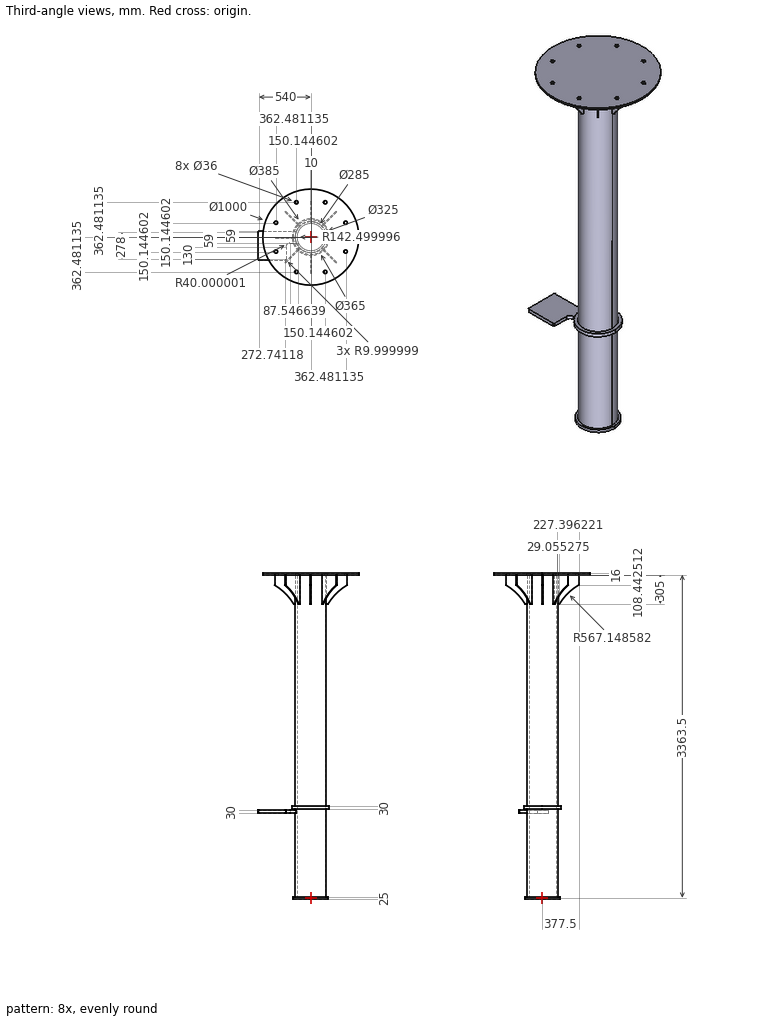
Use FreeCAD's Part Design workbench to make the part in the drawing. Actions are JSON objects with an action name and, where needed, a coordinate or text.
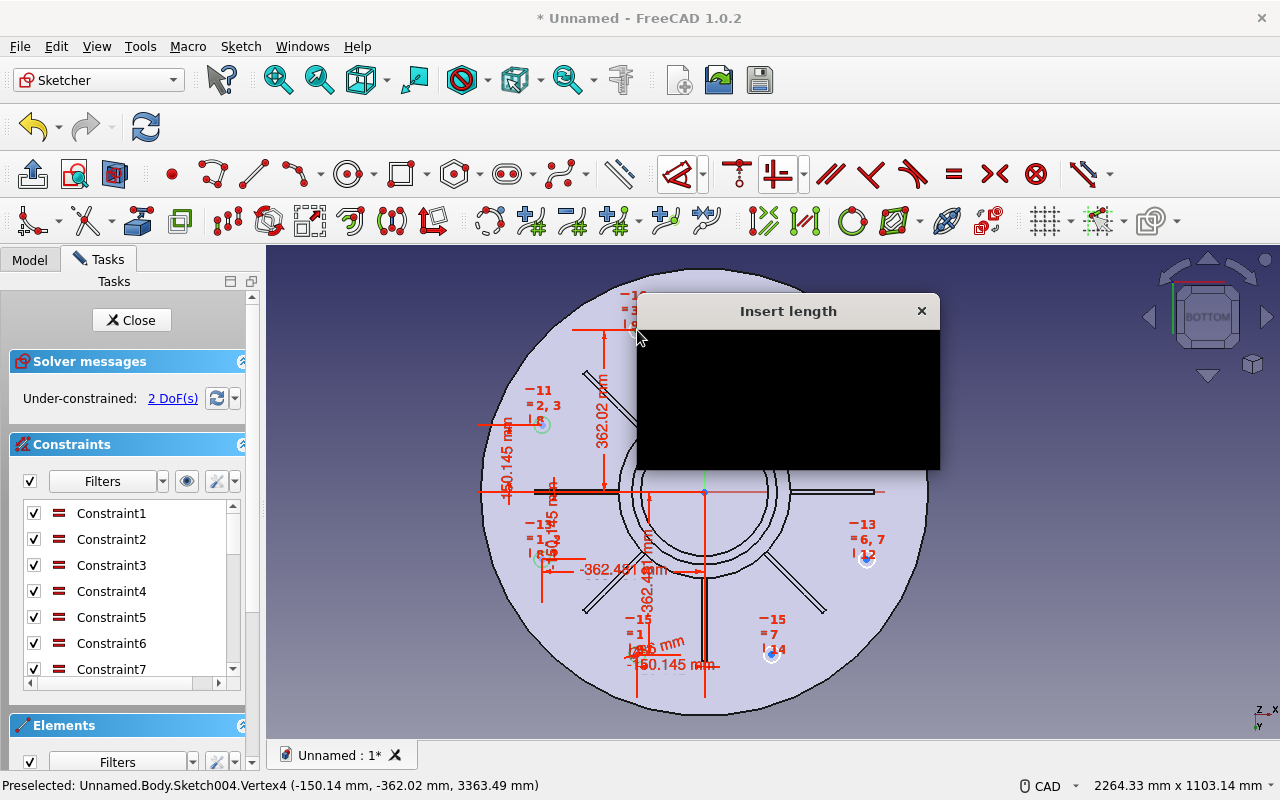
{"action": "type", "text": "362.481135"}
{"action": "key", "text": "Return"}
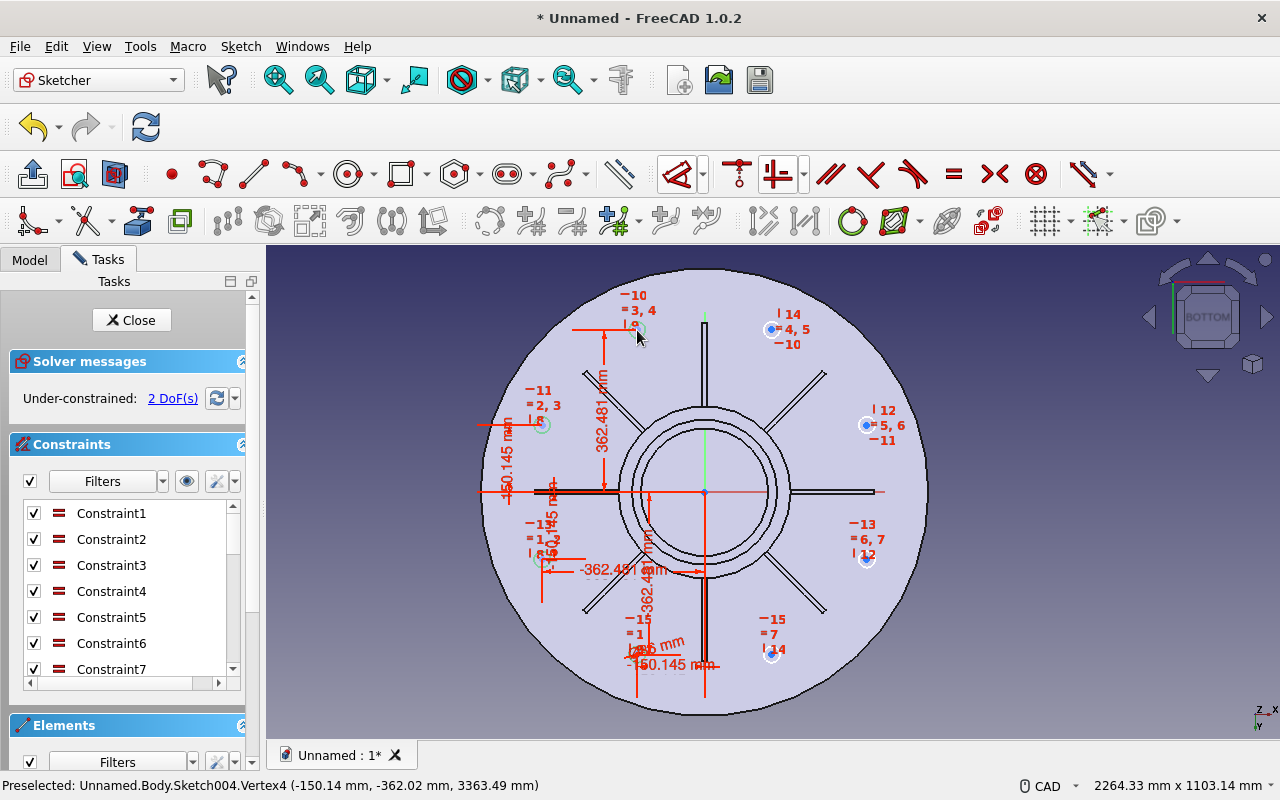
{"action": "left_click", "coordinate": [772, 330]}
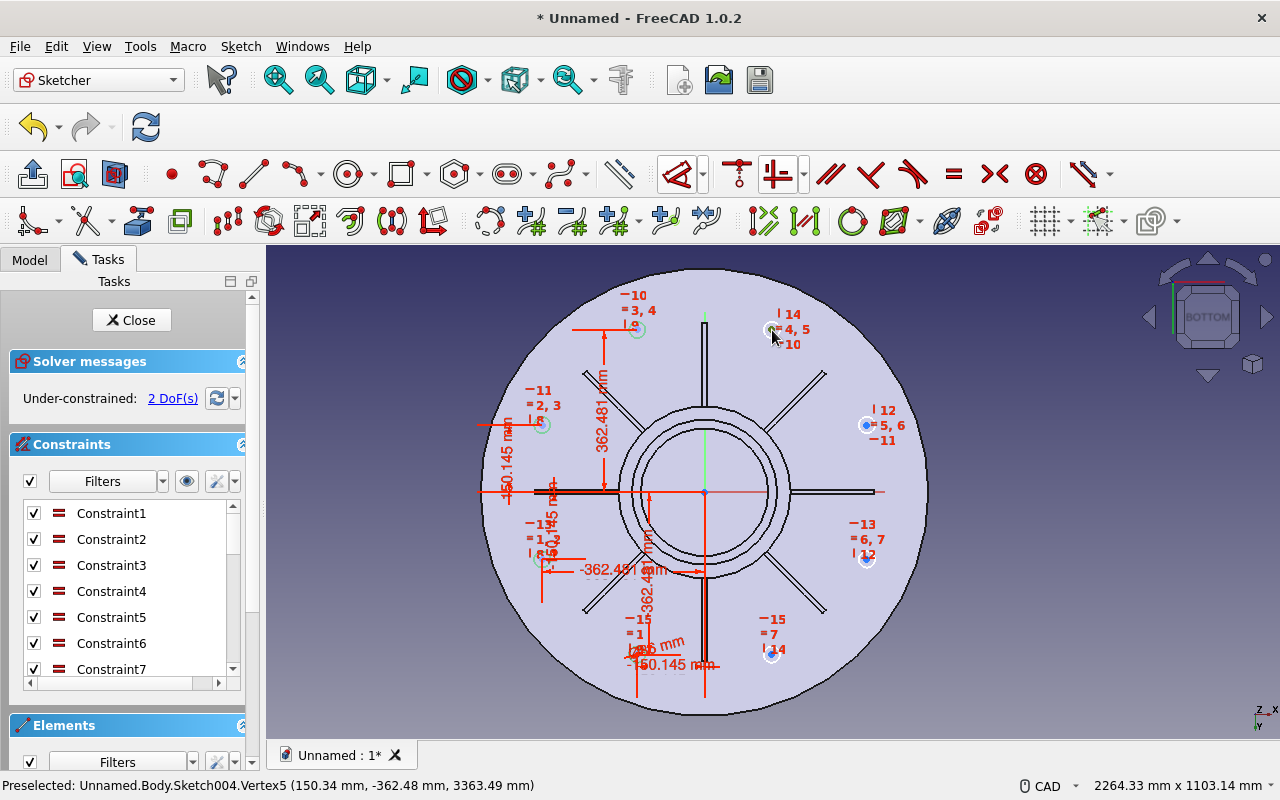
{"action": "left_click", "coordinate": [702, 174]}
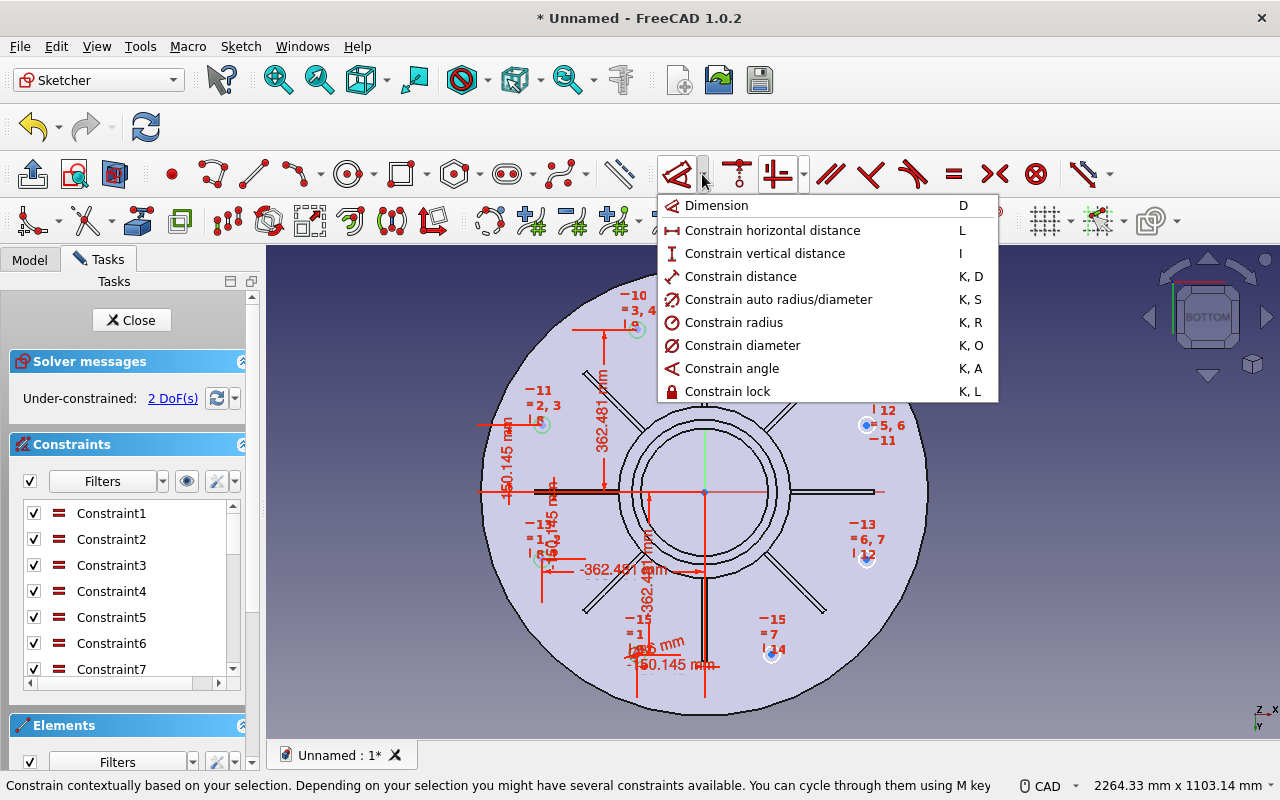
{"action": "left_click", "coordinate": [828, 230]}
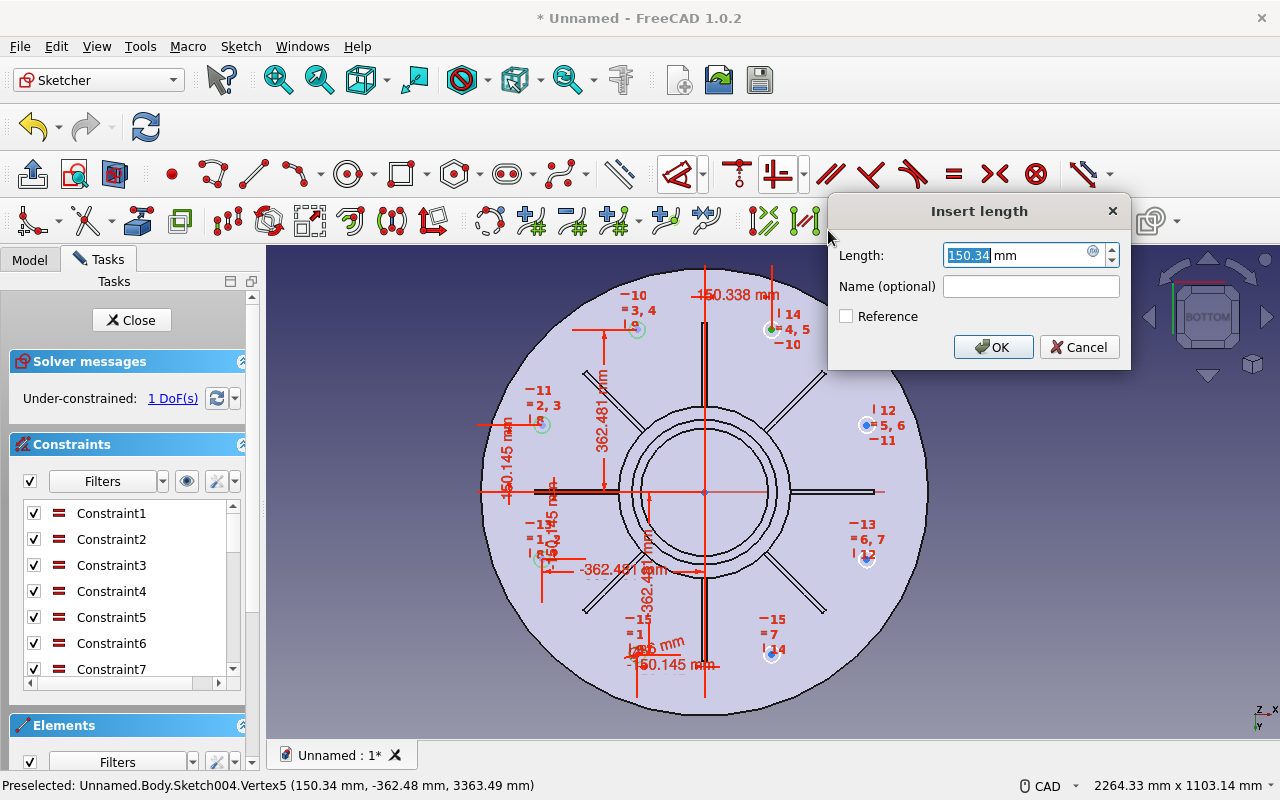
{"action": "type", "text": "150.144602"}
{"action": "key", "text": "Return"}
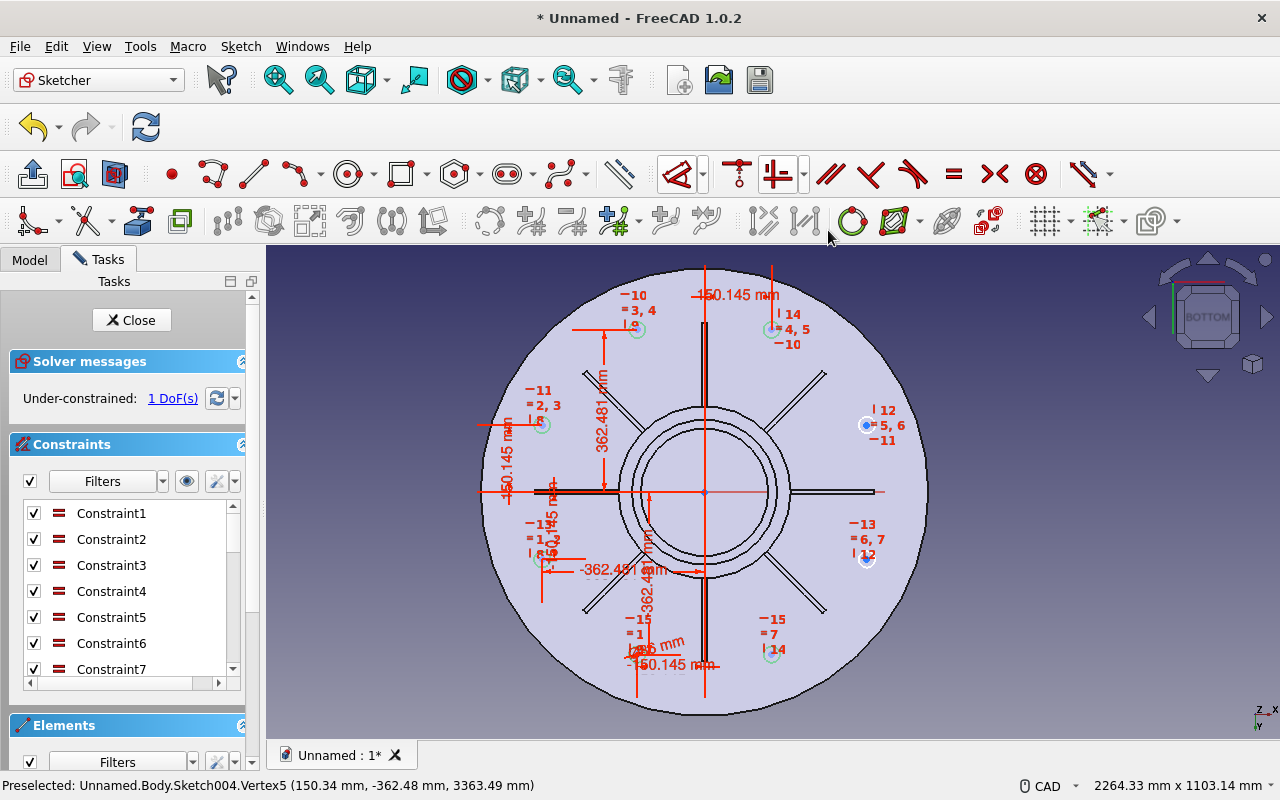
{"action": "left_click", "coordinate": [867, 425]}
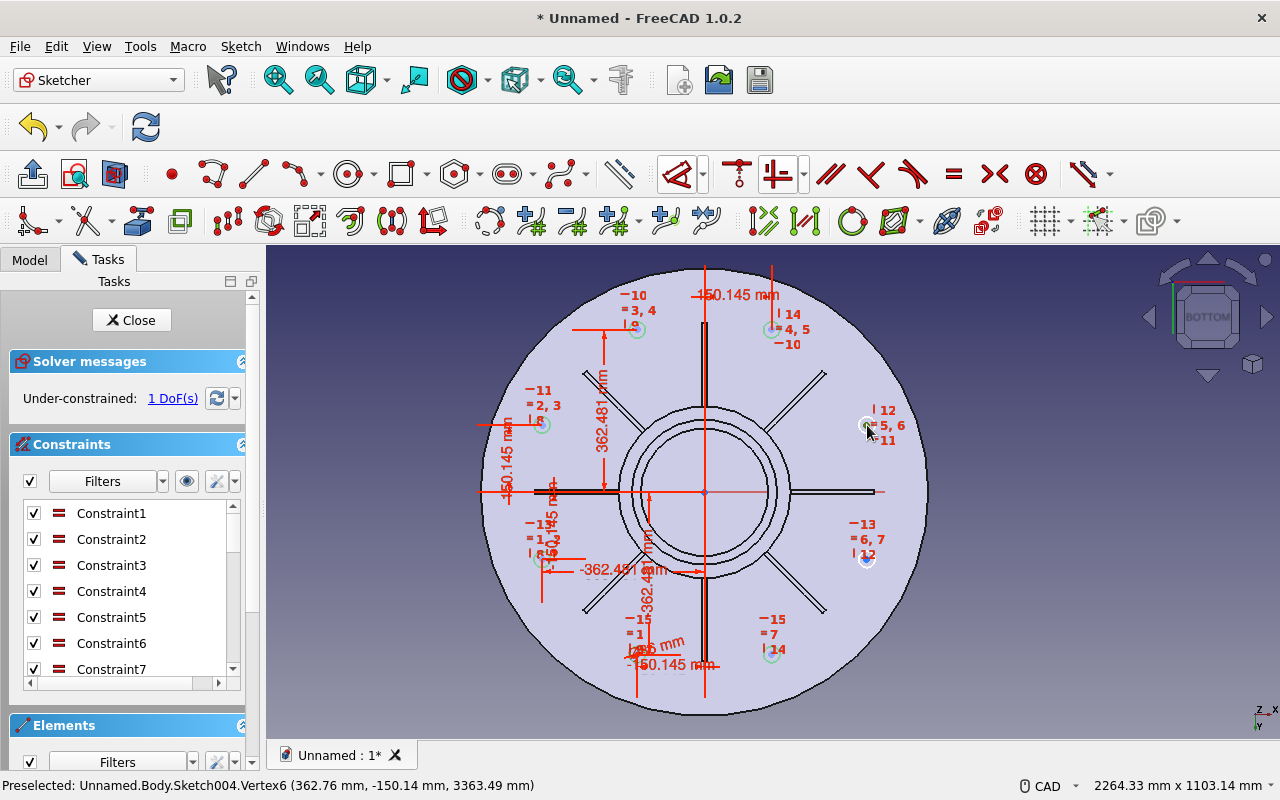
{"action": "key", "text": "l"}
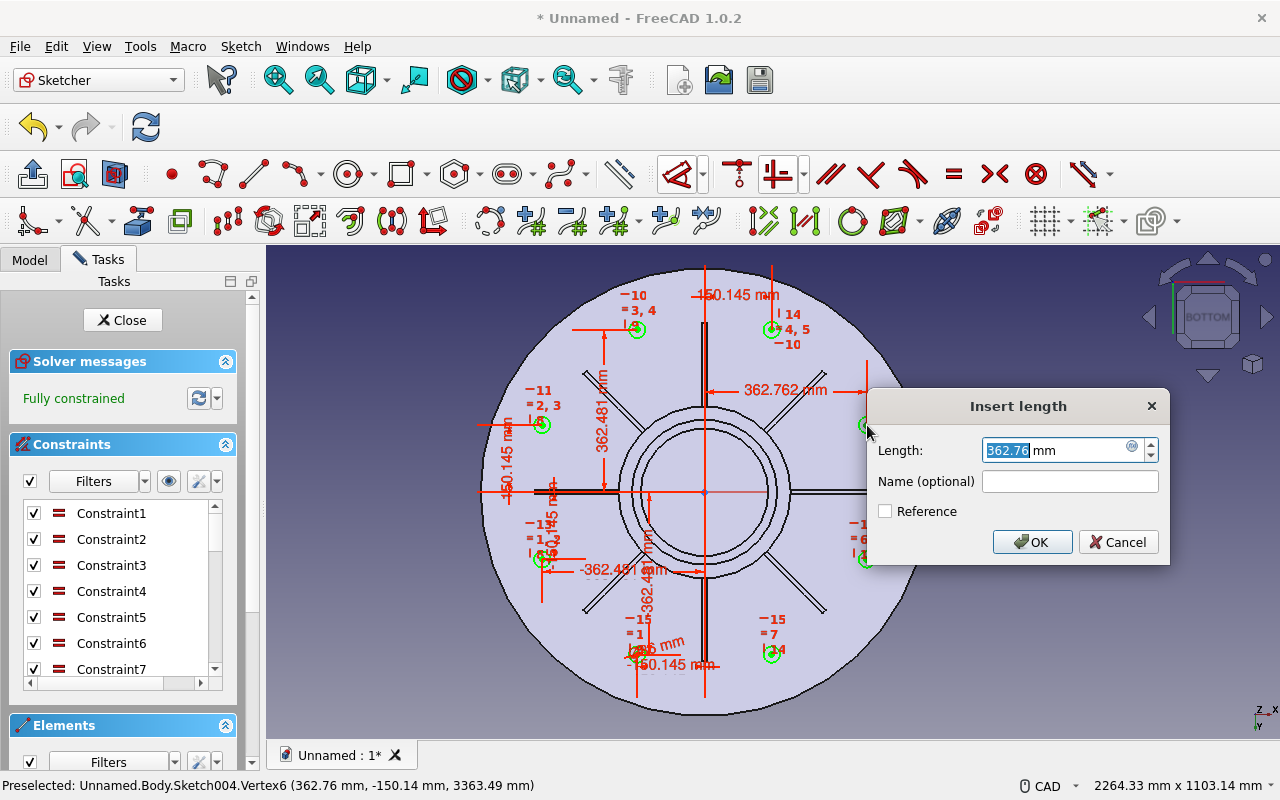
{"action": "type", "text": "362.481135"}
{"action": "key", "text": "Return"}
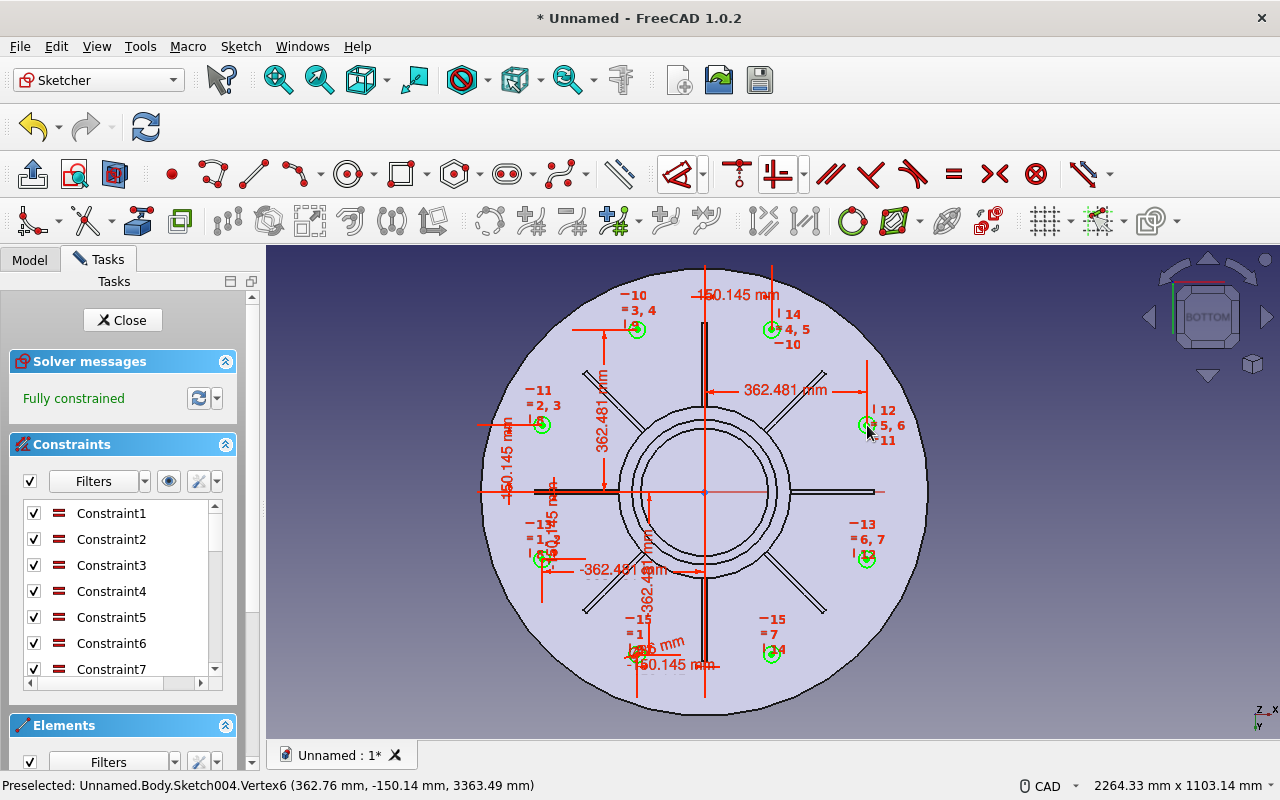
{"action": "left_click", "coordinate": [123, 320]}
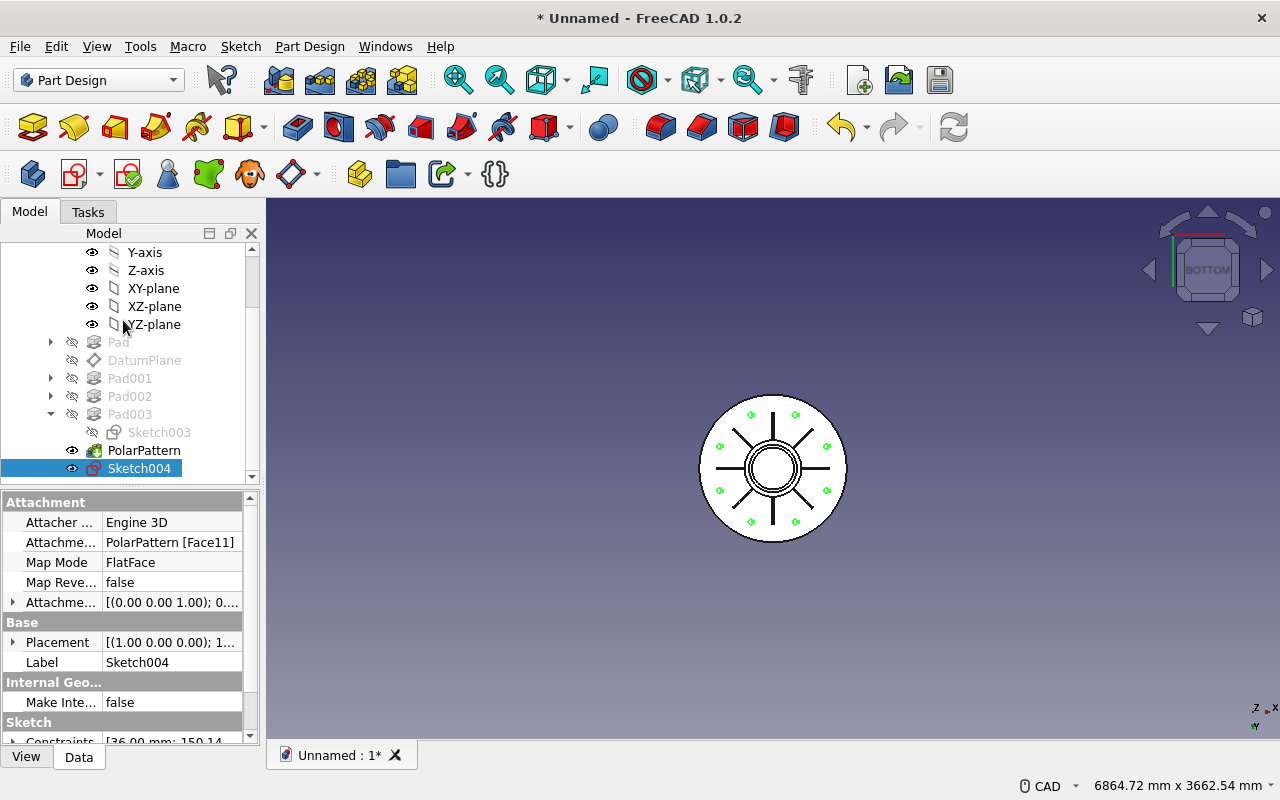
{"action": "left_click", "coordinate": [298, 128]}